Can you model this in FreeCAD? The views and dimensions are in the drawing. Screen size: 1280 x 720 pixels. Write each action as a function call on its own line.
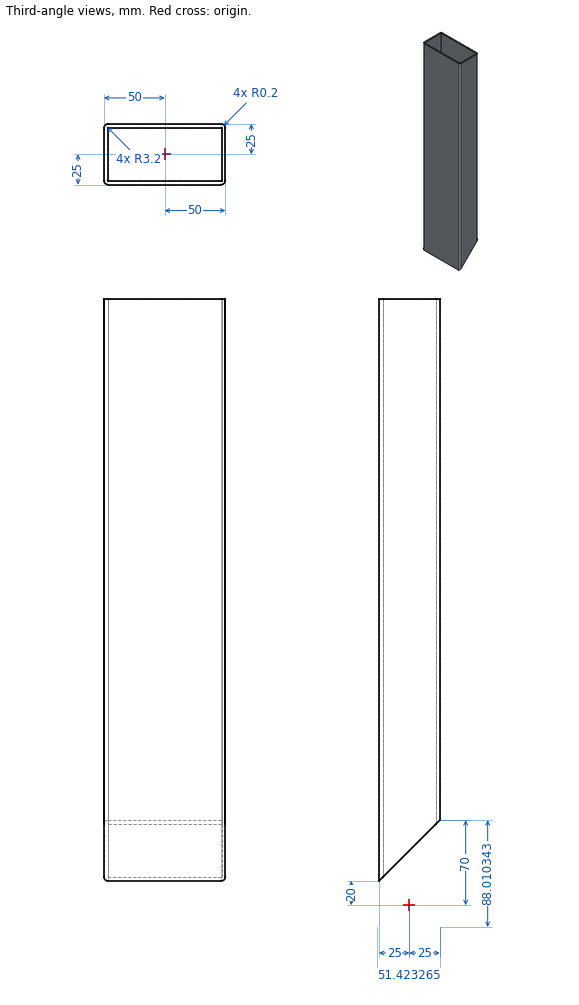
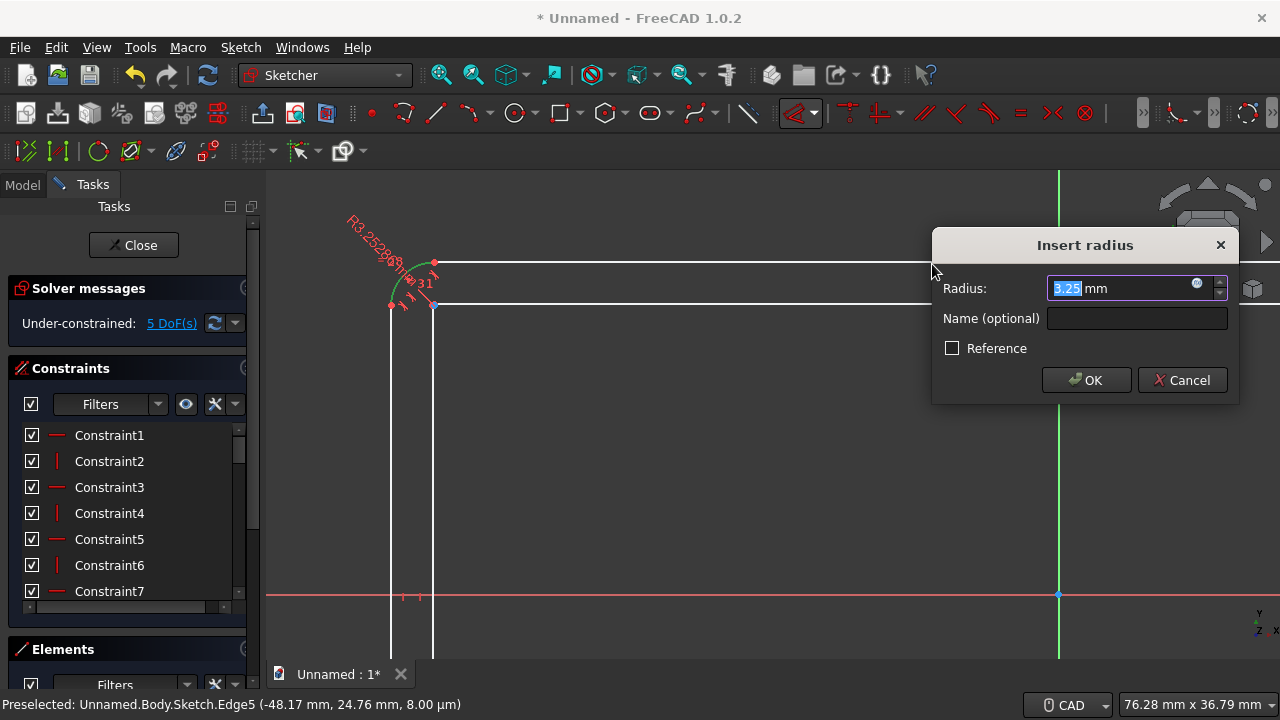
text(3.2)
key(Return)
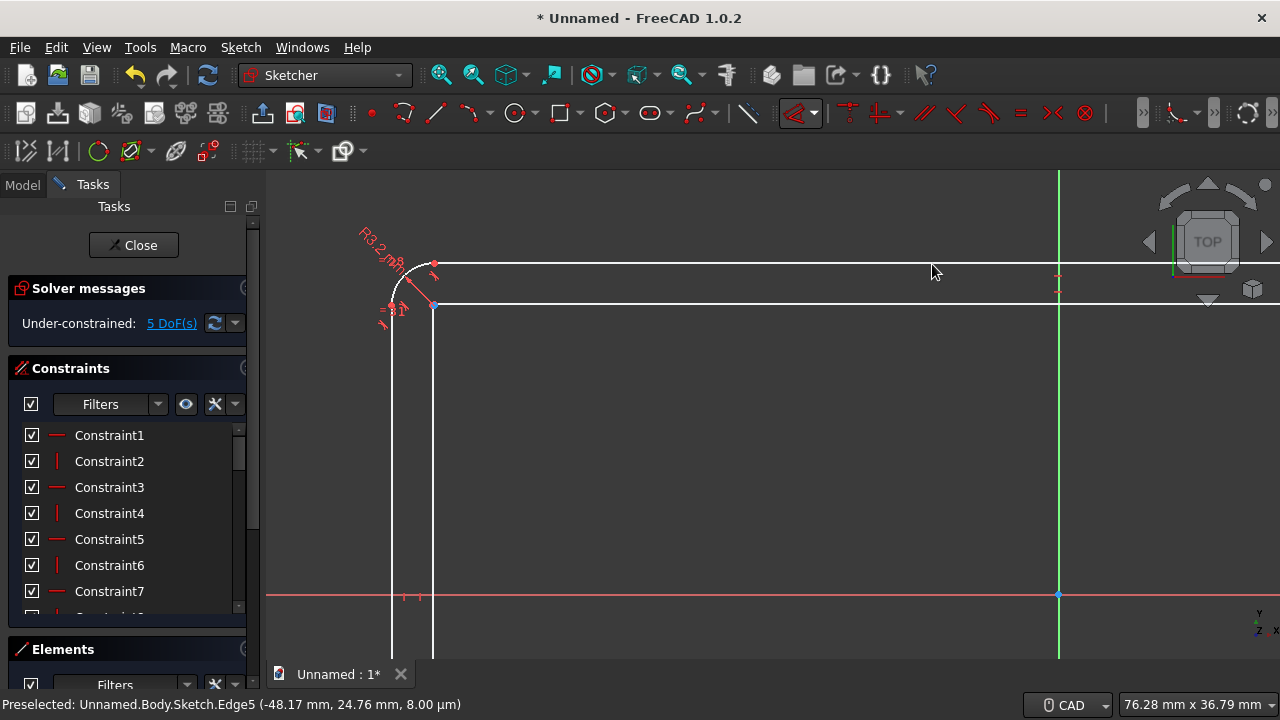
scroll(415, 268, down, 4)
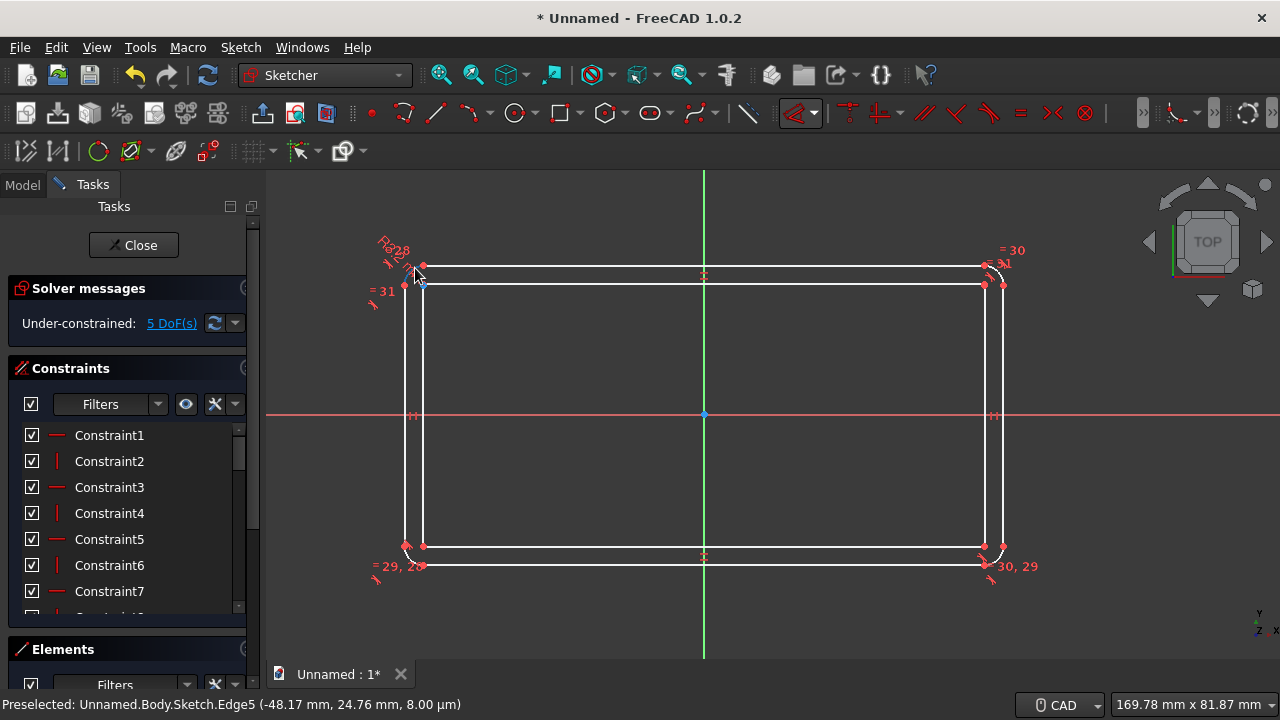
scroll(985, 285, up, 18)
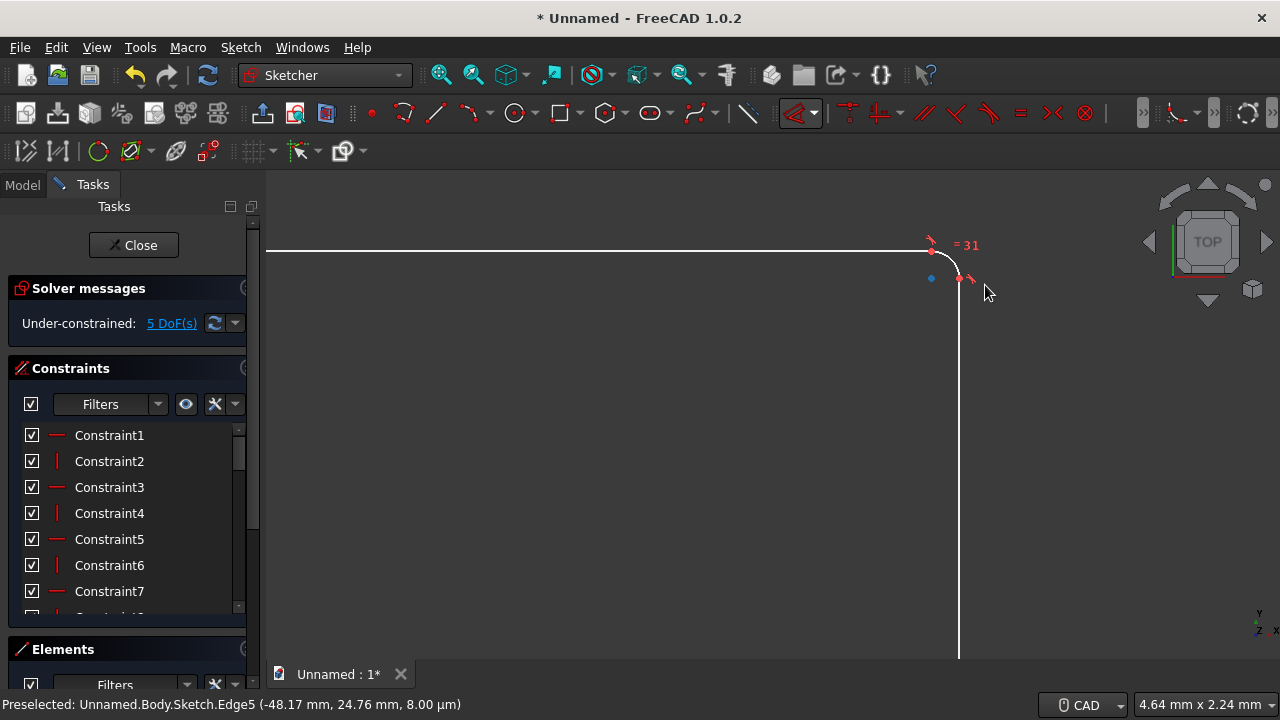
click(951, 260)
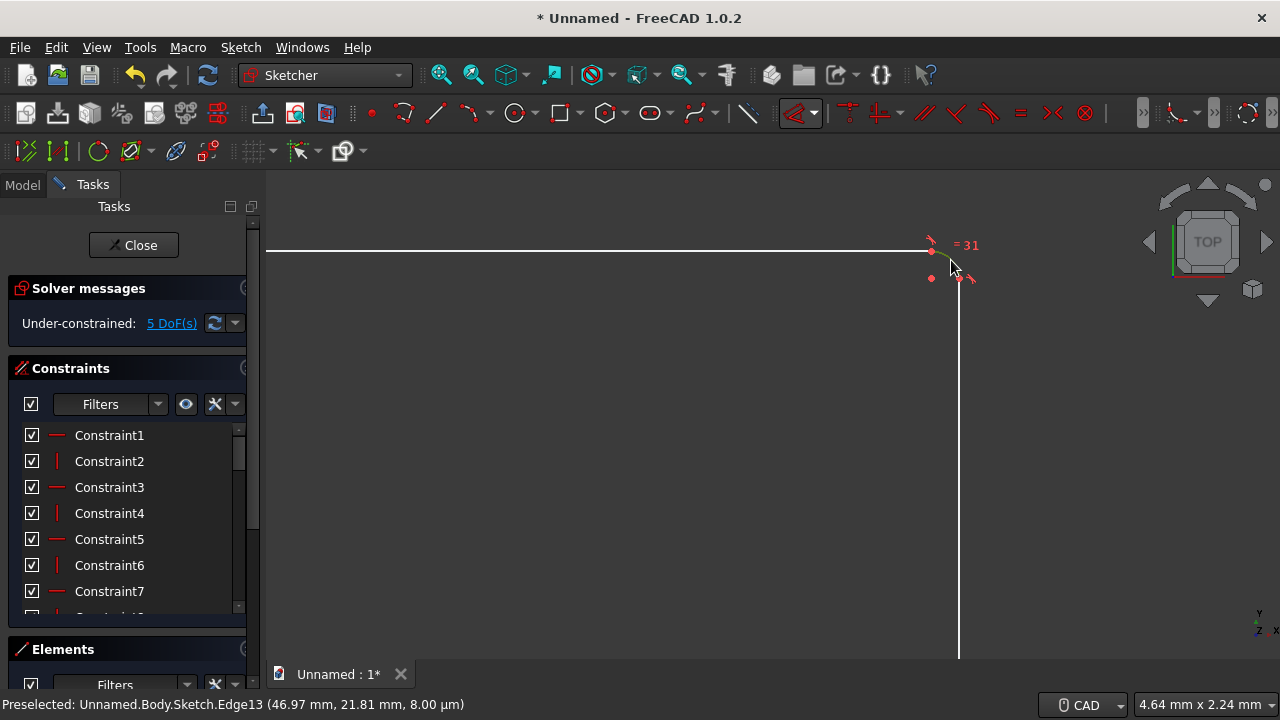
click(816, 114)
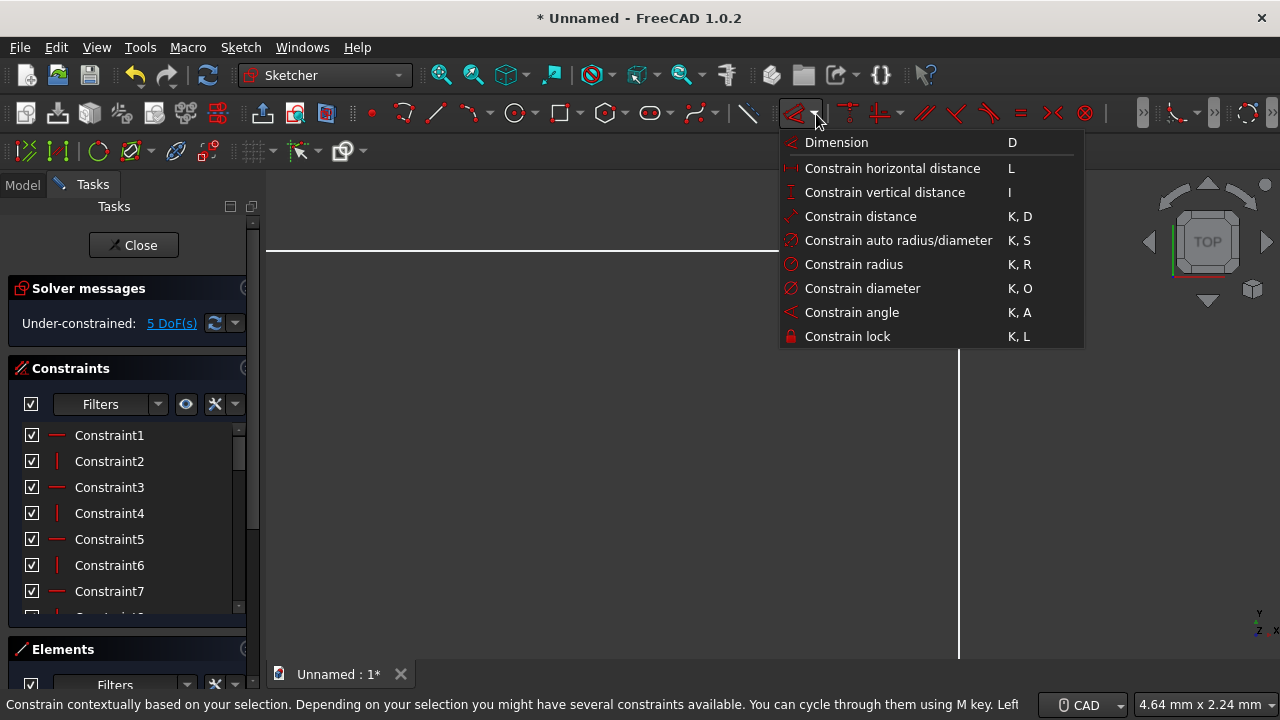
click(932, 264)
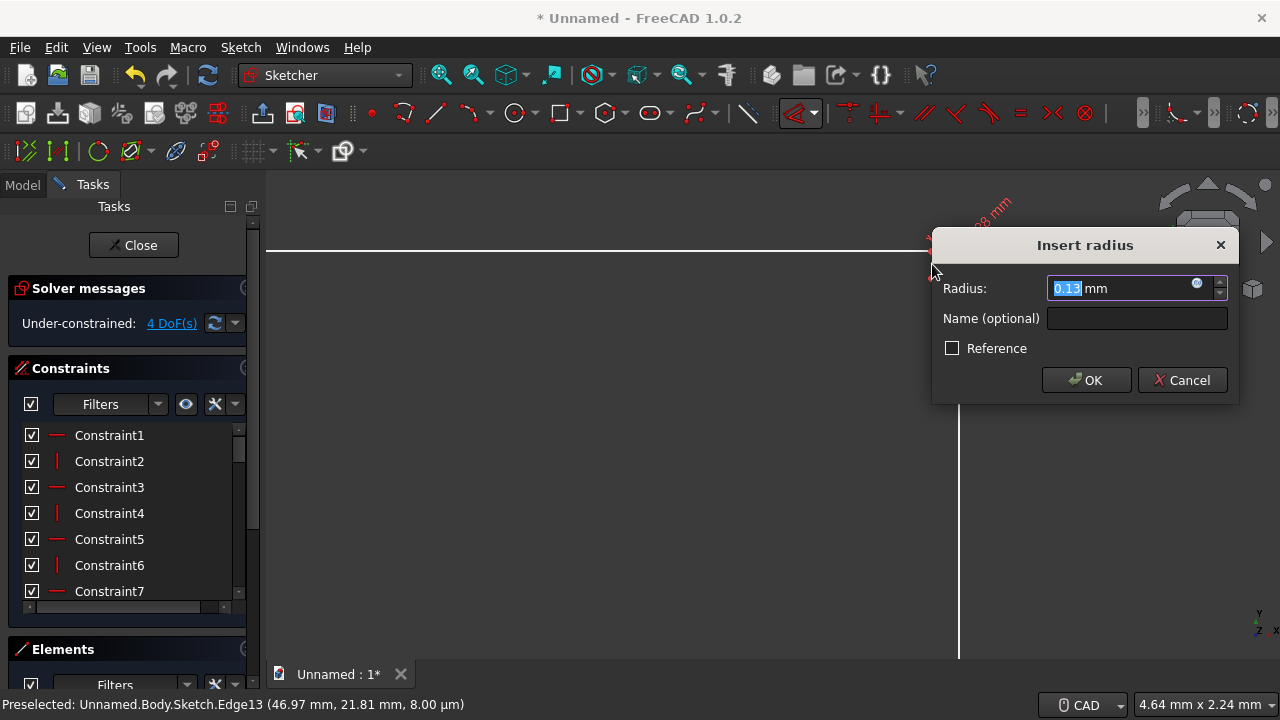
text(0.2)
key(Return)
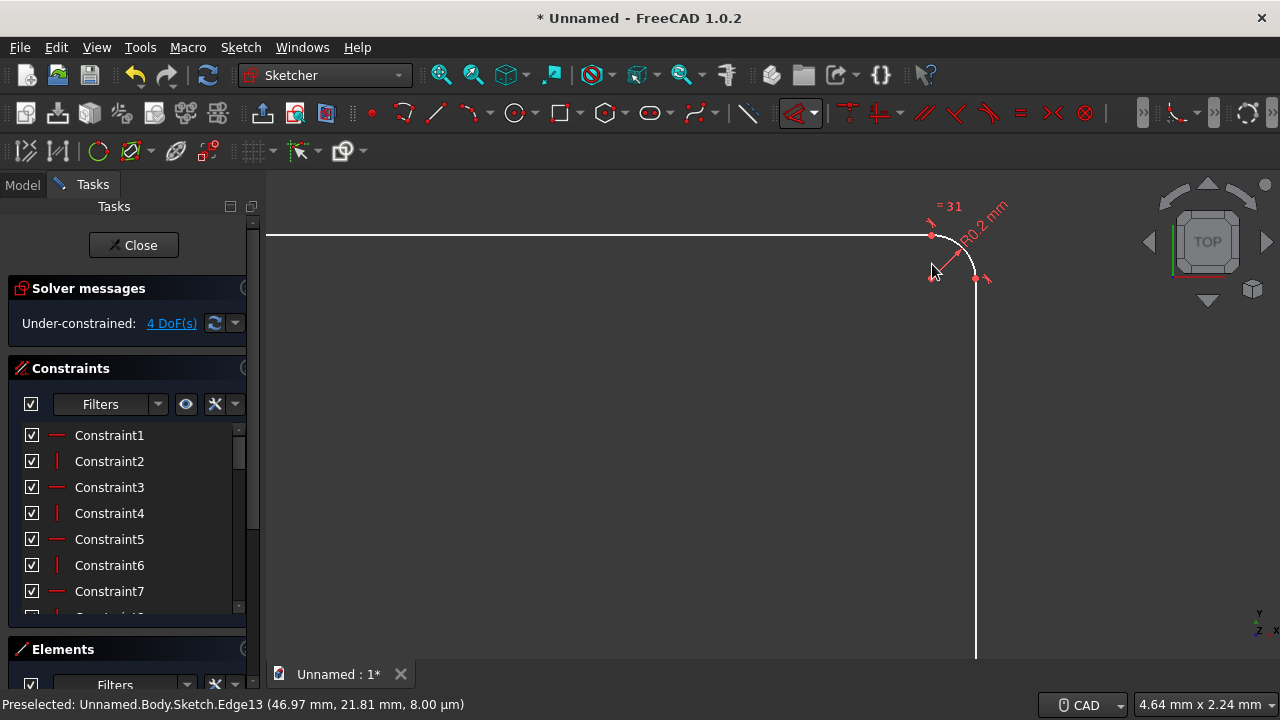
scroll(1050, 255, down, 17)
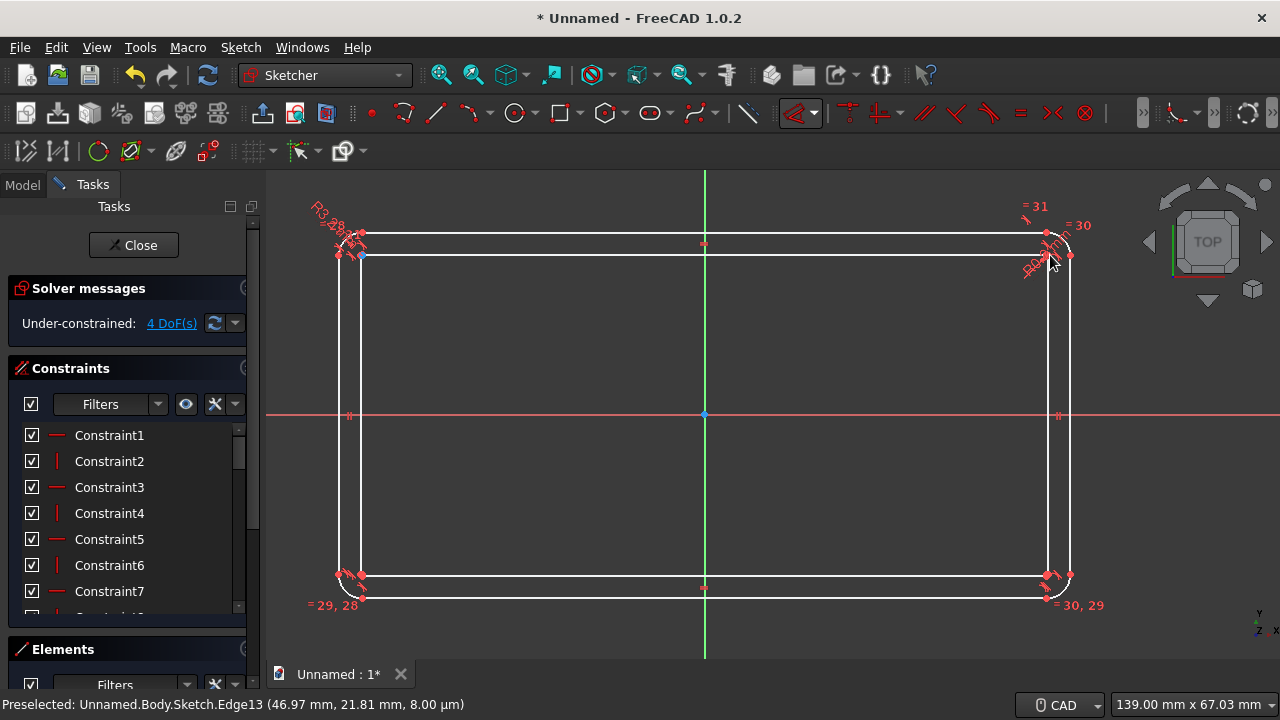
click(1047, 233)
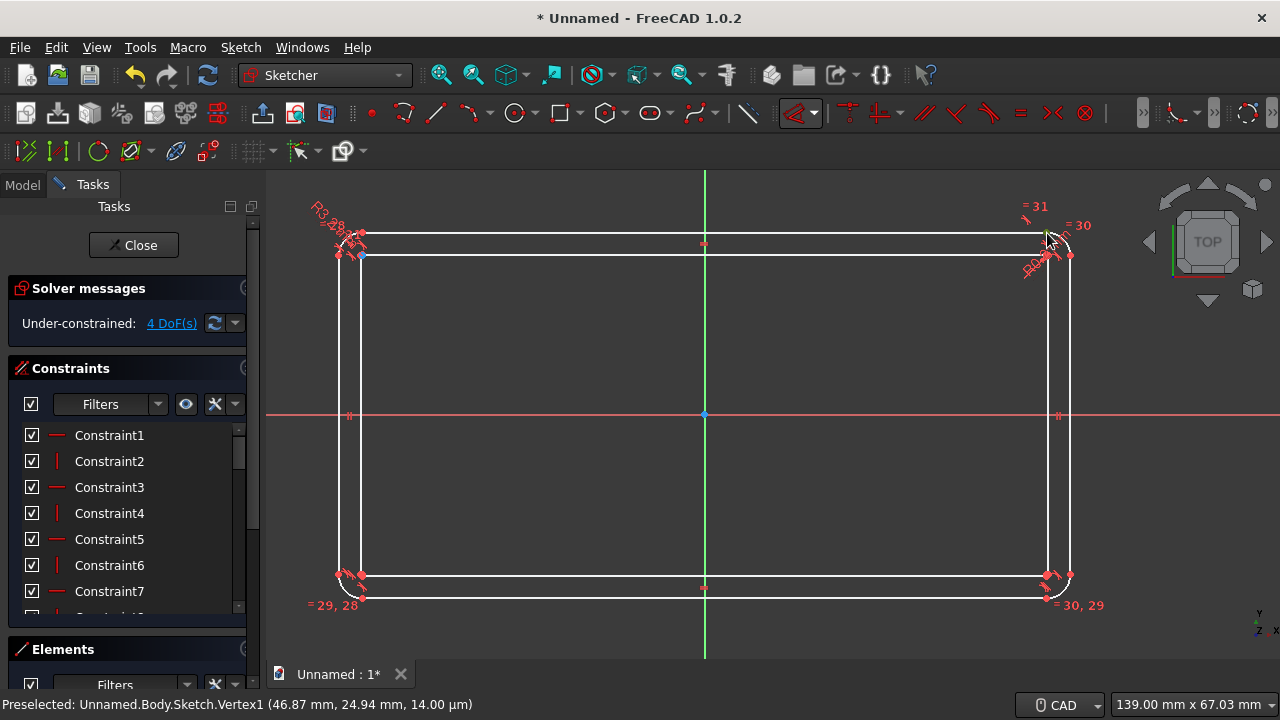
click(816, 114)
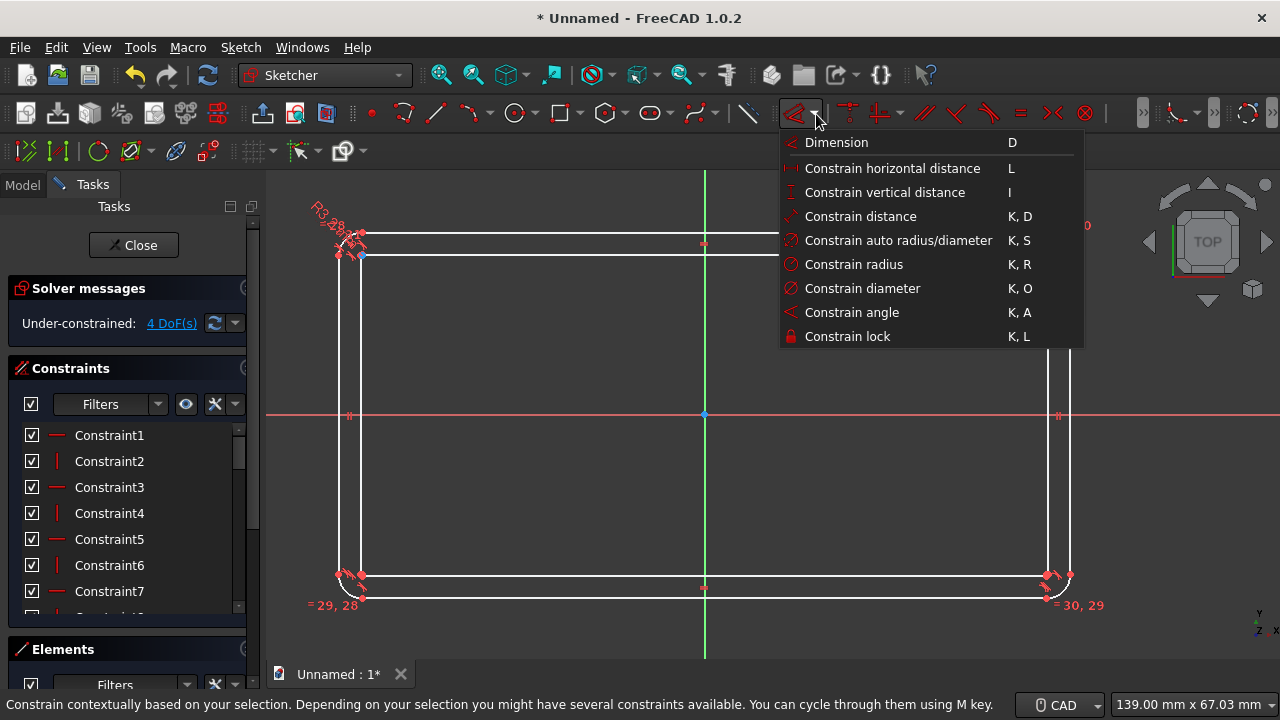
click(932, 192)